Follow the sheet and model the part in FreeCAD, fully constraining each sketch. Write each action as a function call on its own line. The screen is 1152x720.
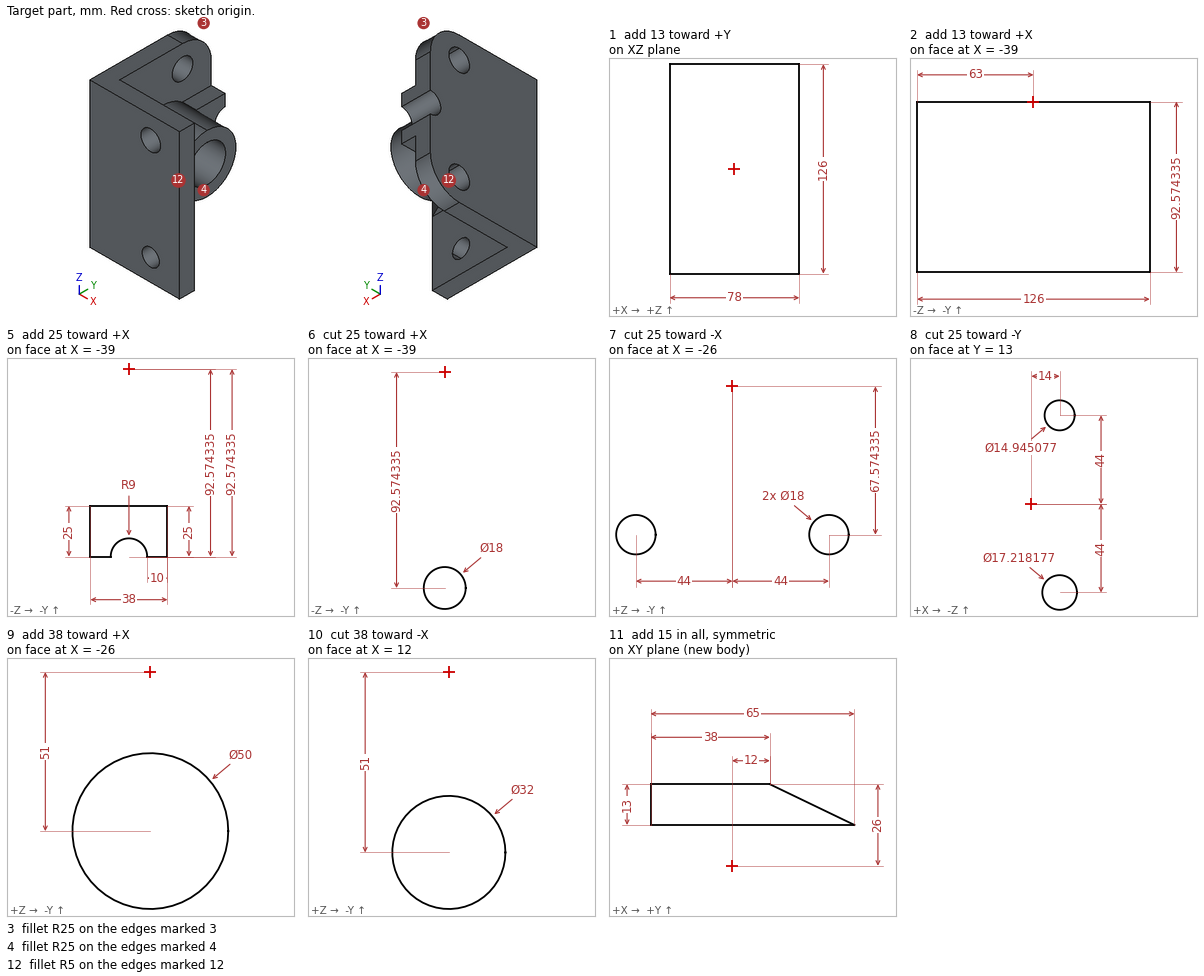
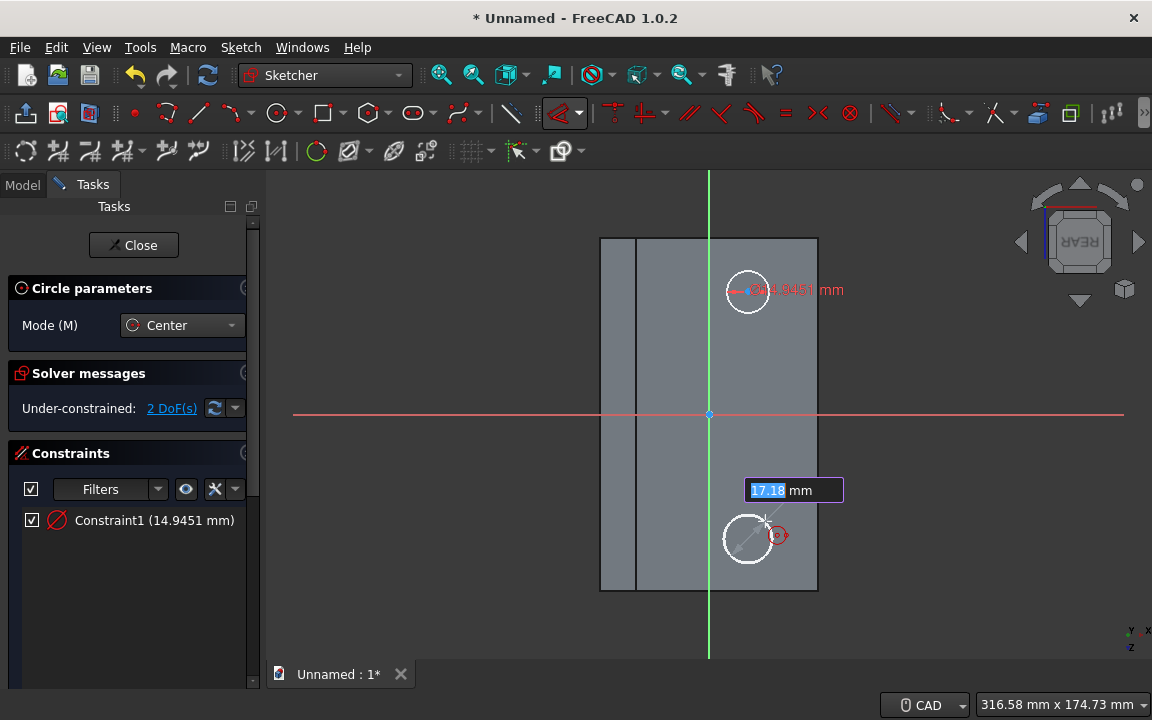
text(17.218177)
key(Return)
key(Escape)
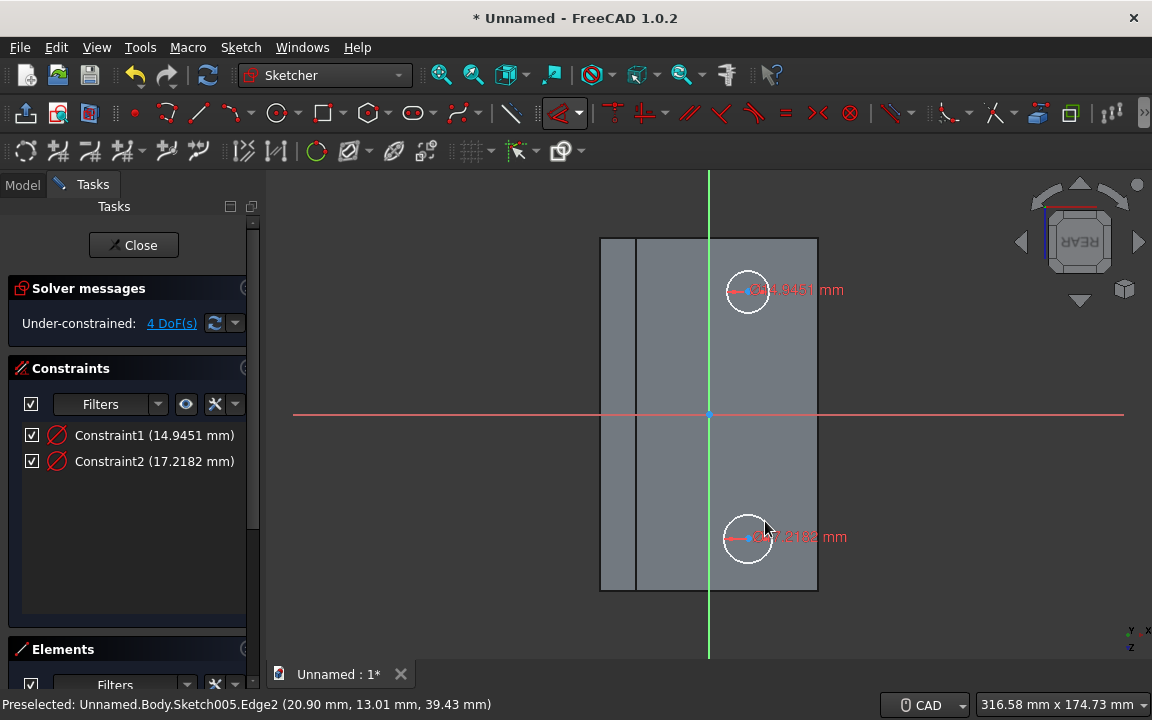
click(748, 292)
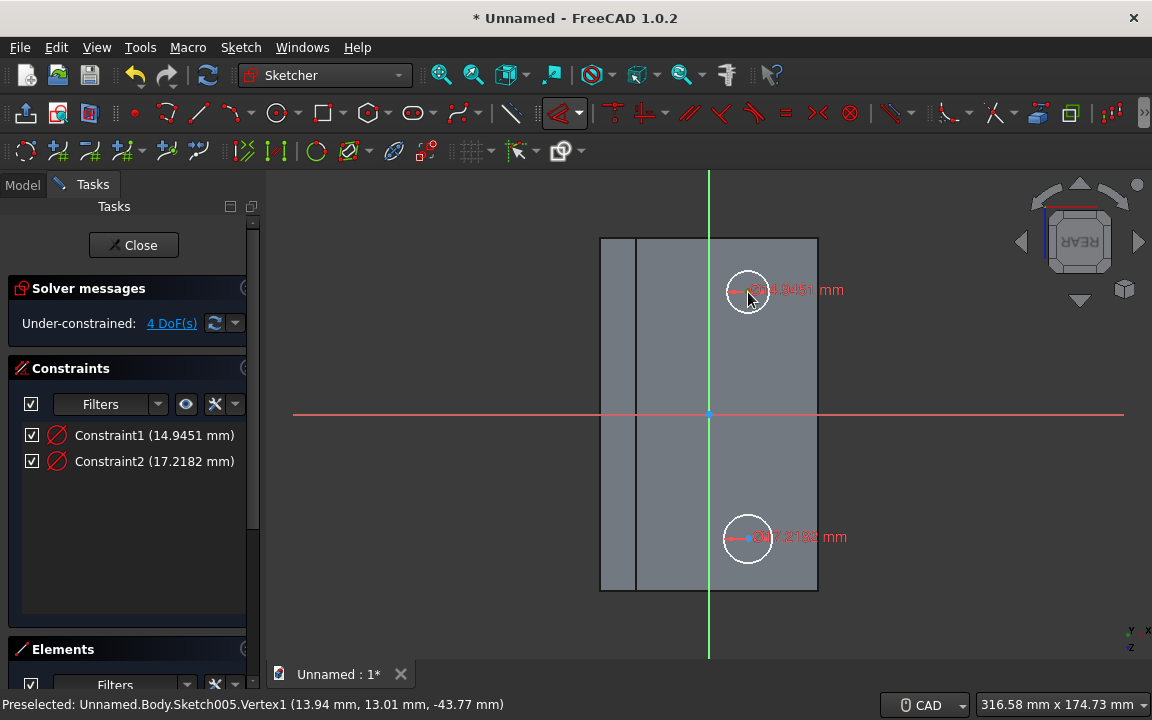
click(748, 539)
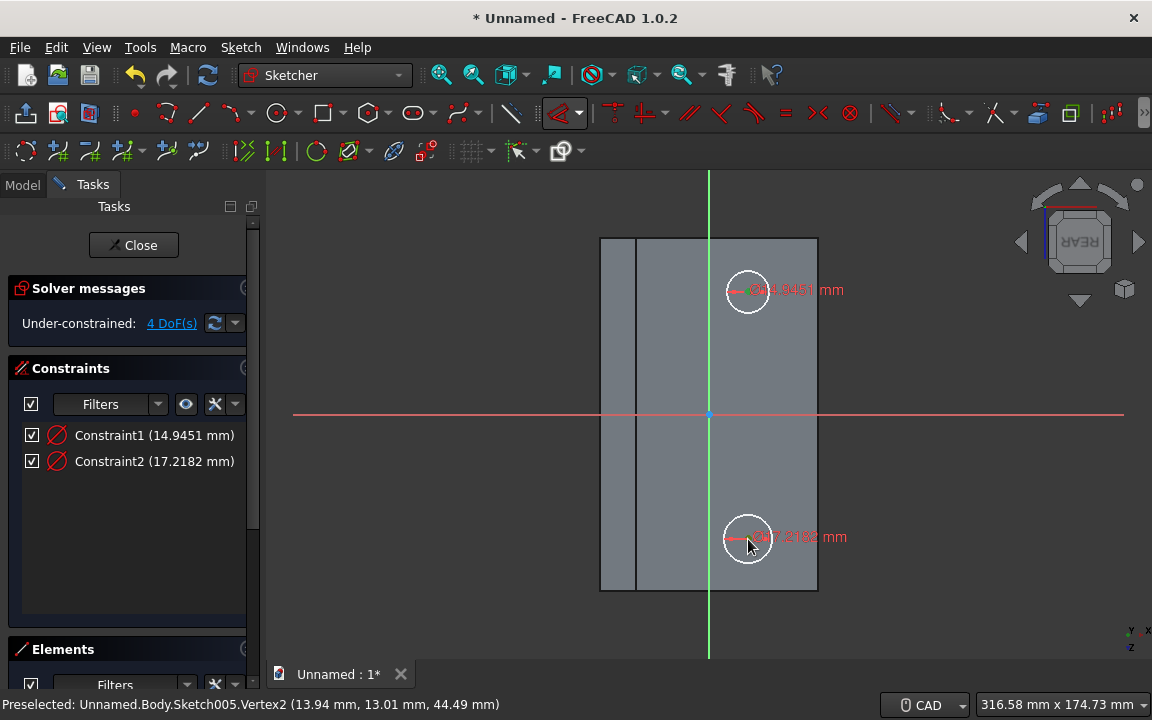
click(668, 114)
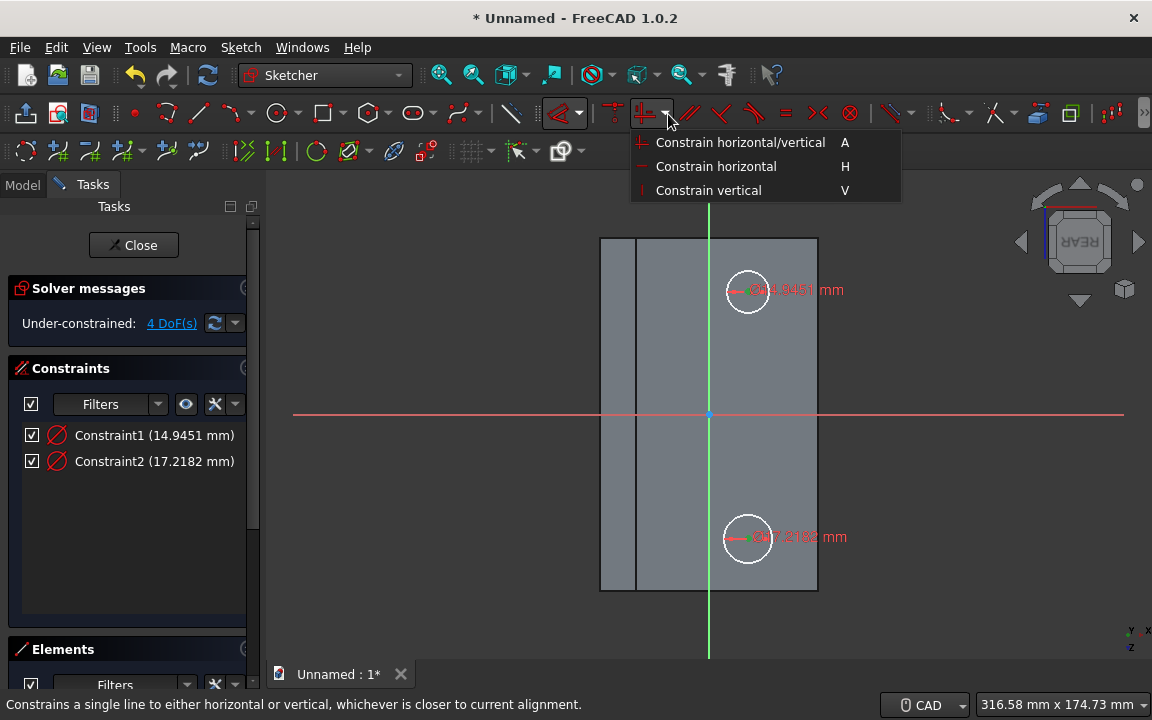
click(766, 190)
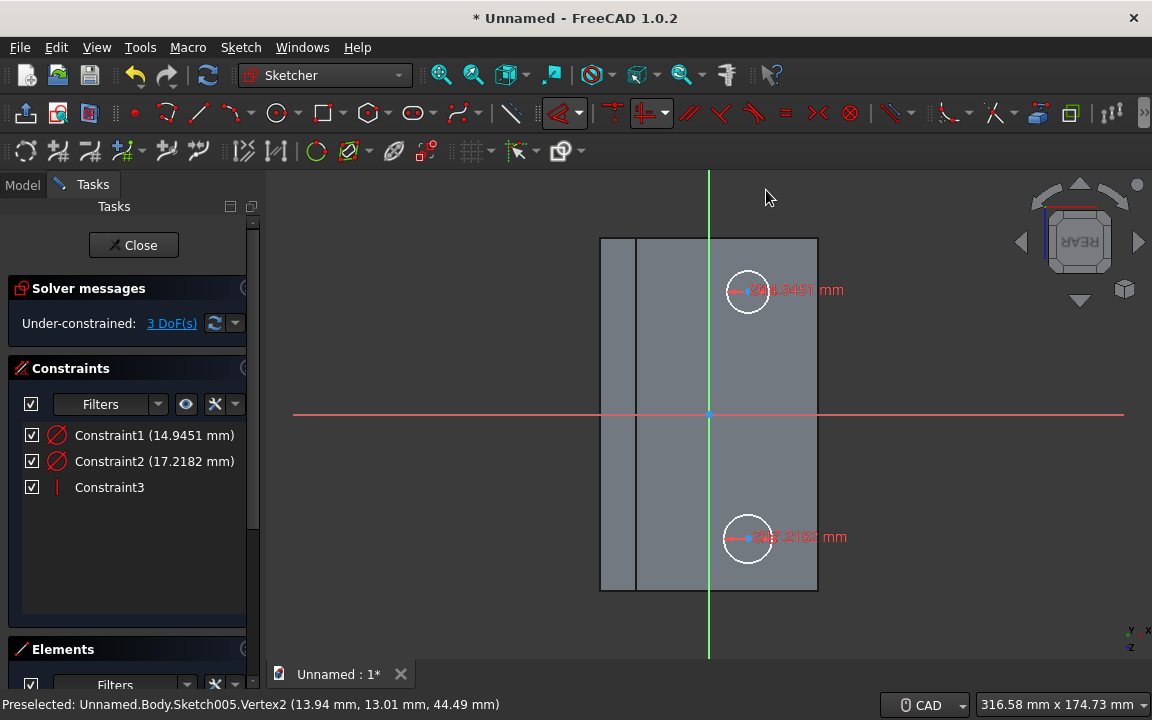
click(748, 292)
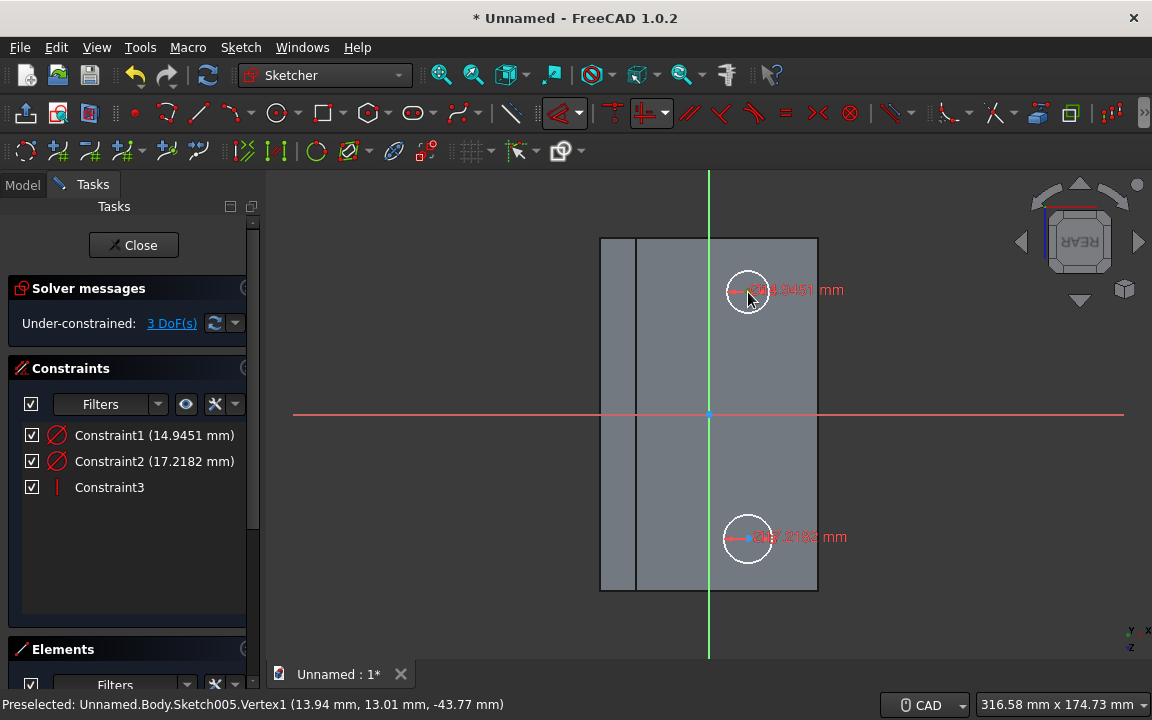
key(l)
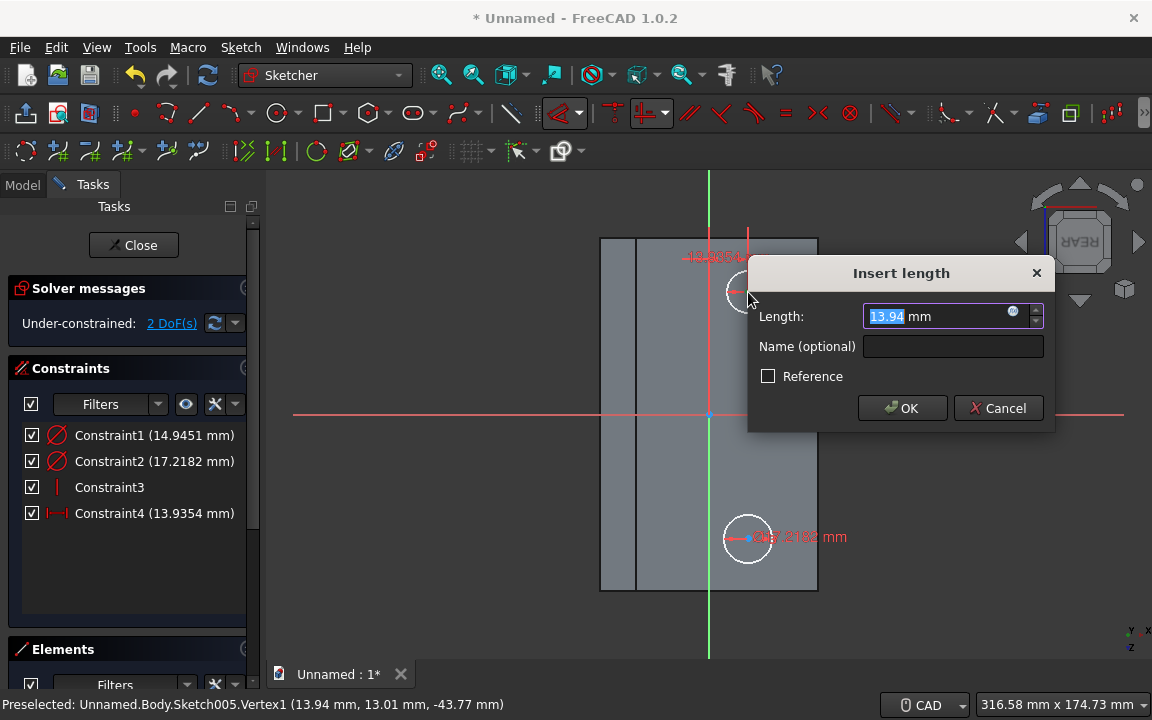
text(14)
key(Return)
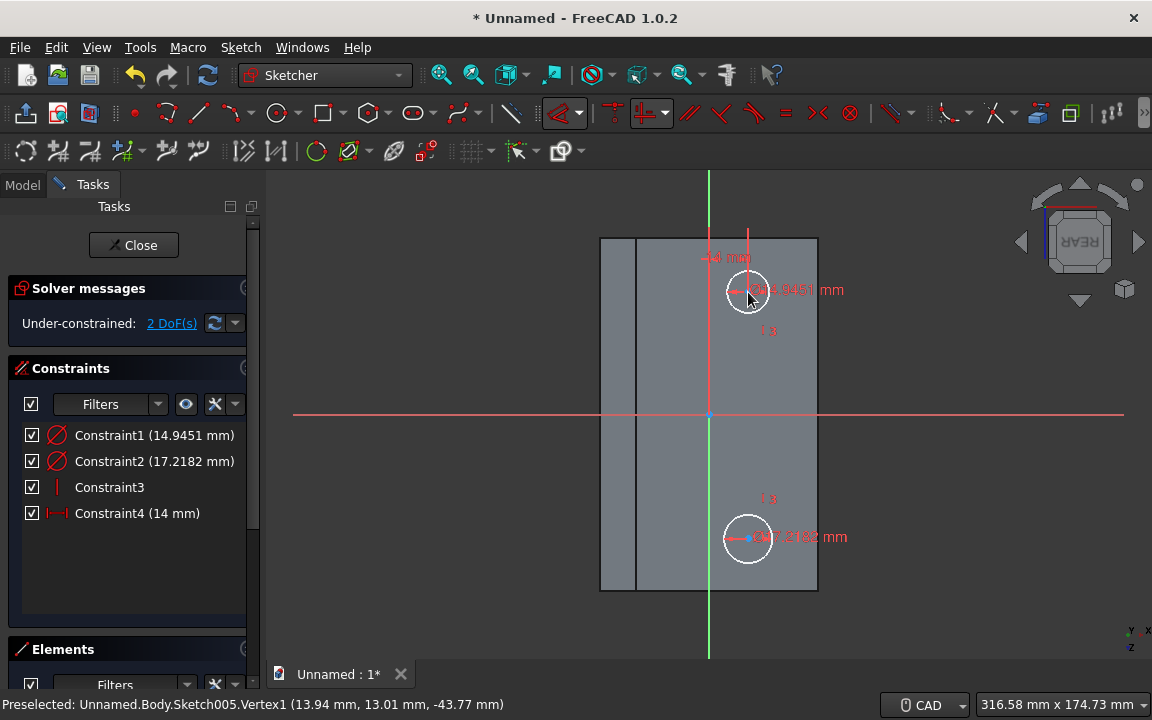
click(748, 292)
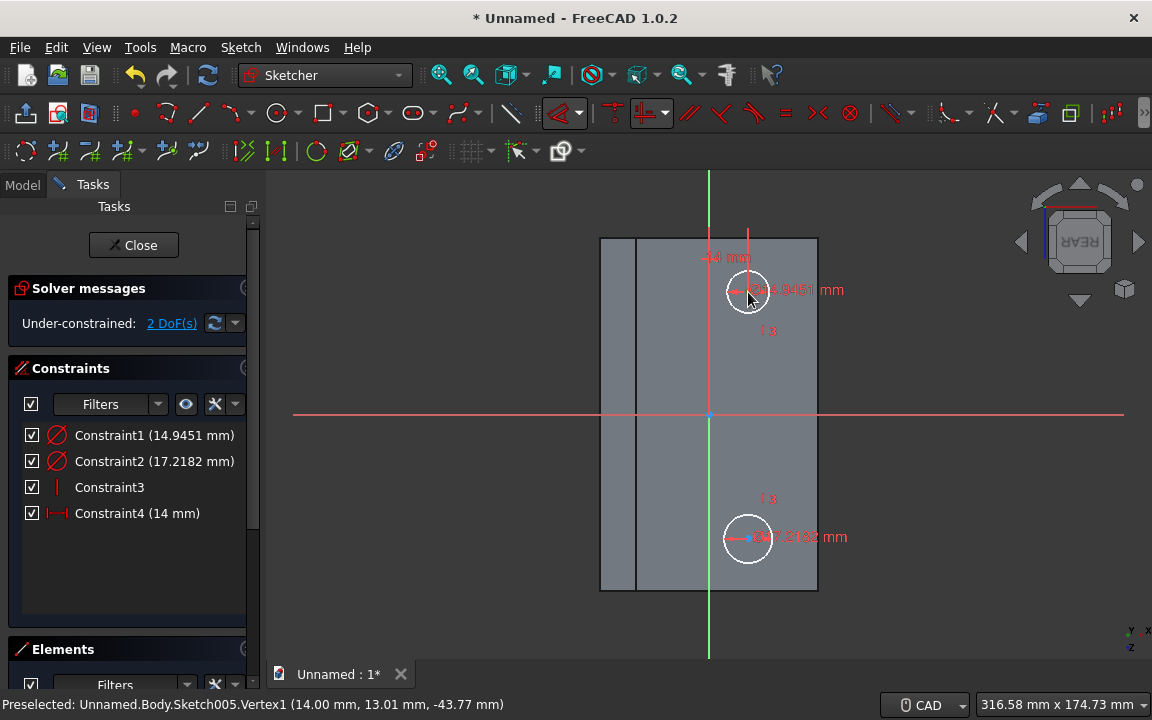
key(i)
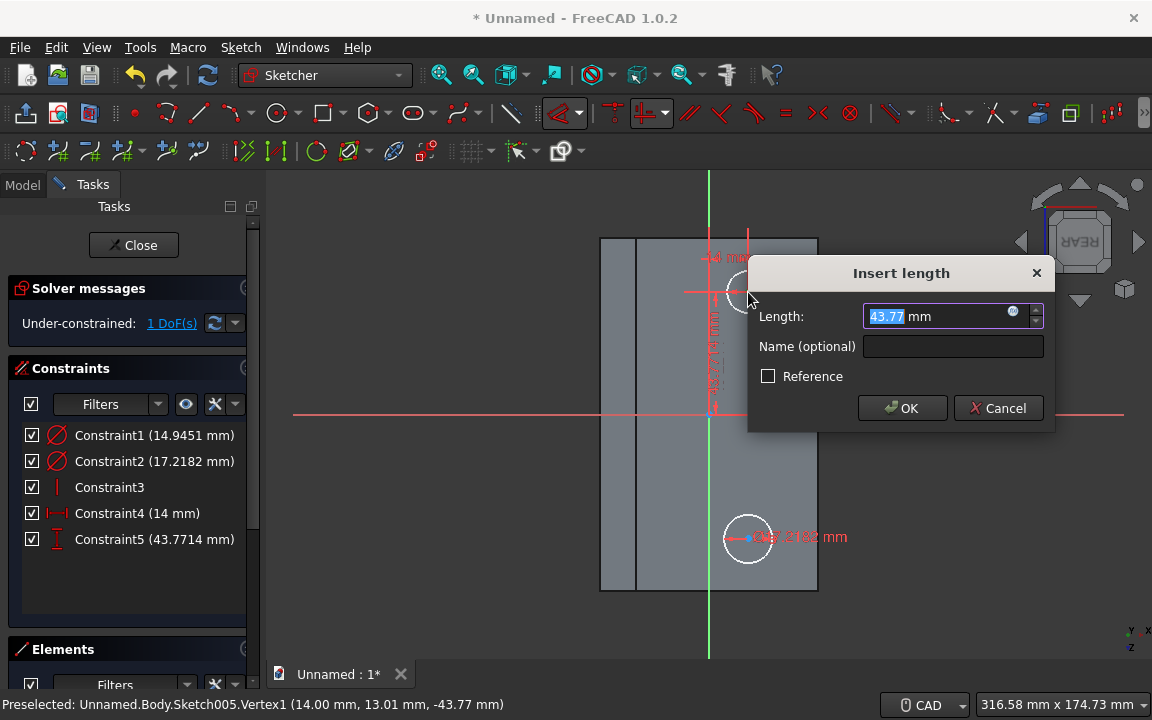
text(44)
key(Return)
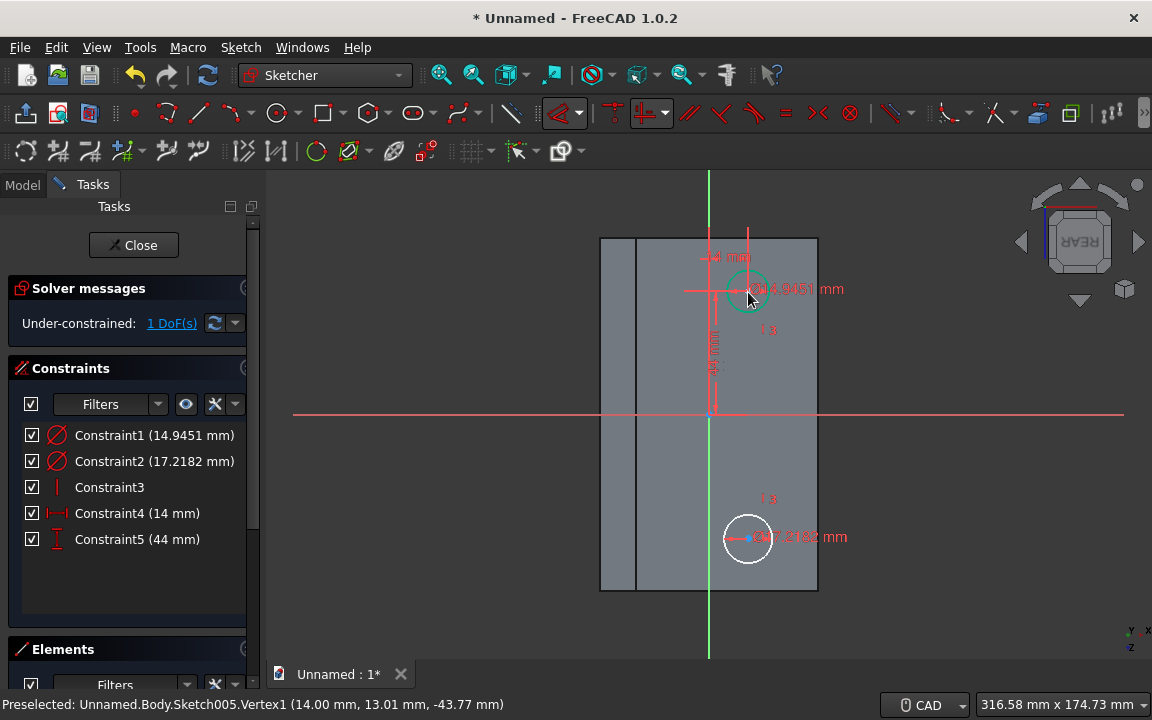
click(748, 539)